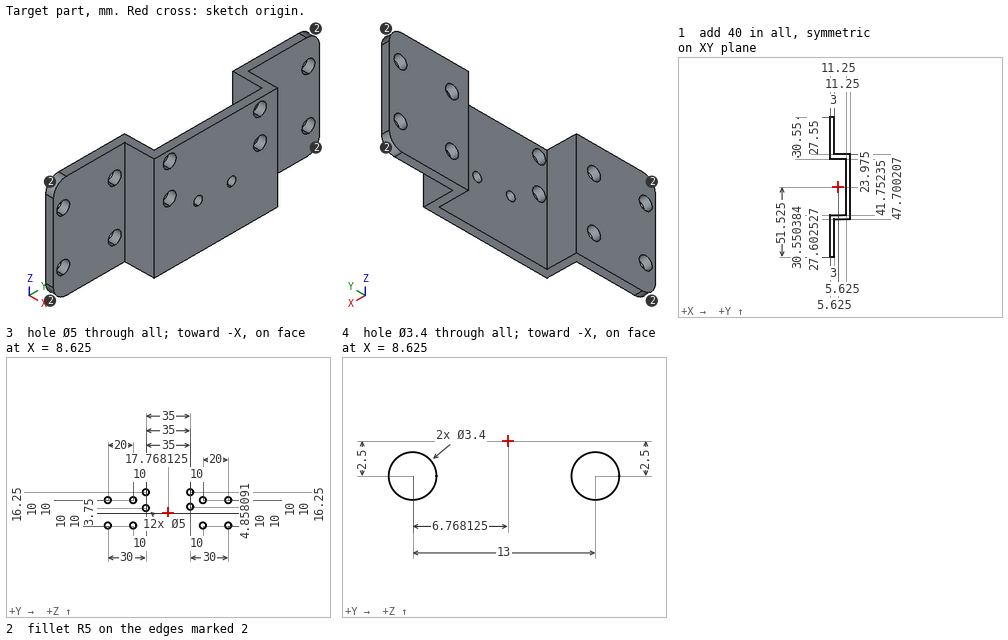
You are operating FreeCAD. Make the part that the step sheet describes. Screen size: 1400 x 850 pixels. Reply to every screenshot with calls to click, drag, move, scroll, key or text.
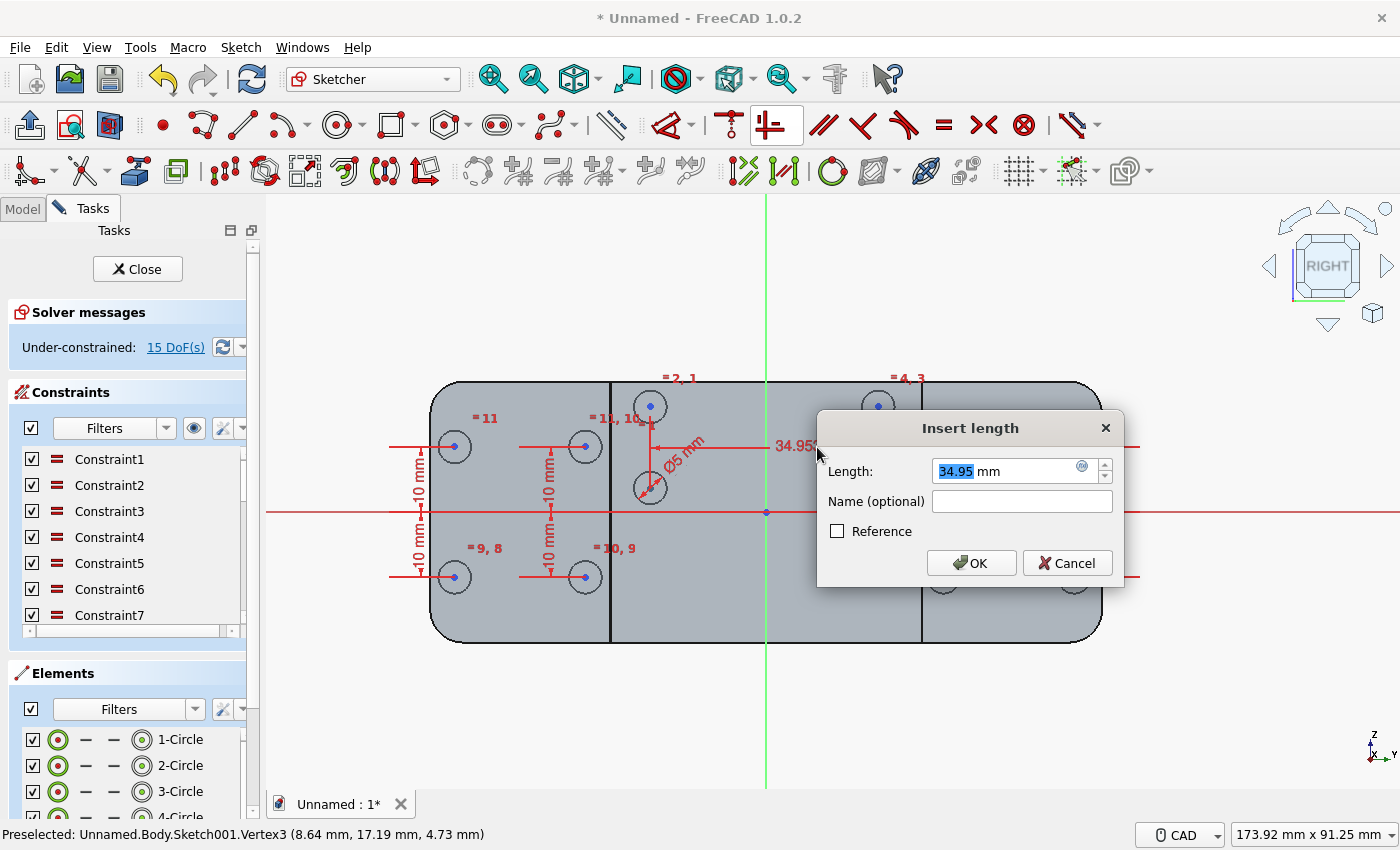
text(35)
key(Return)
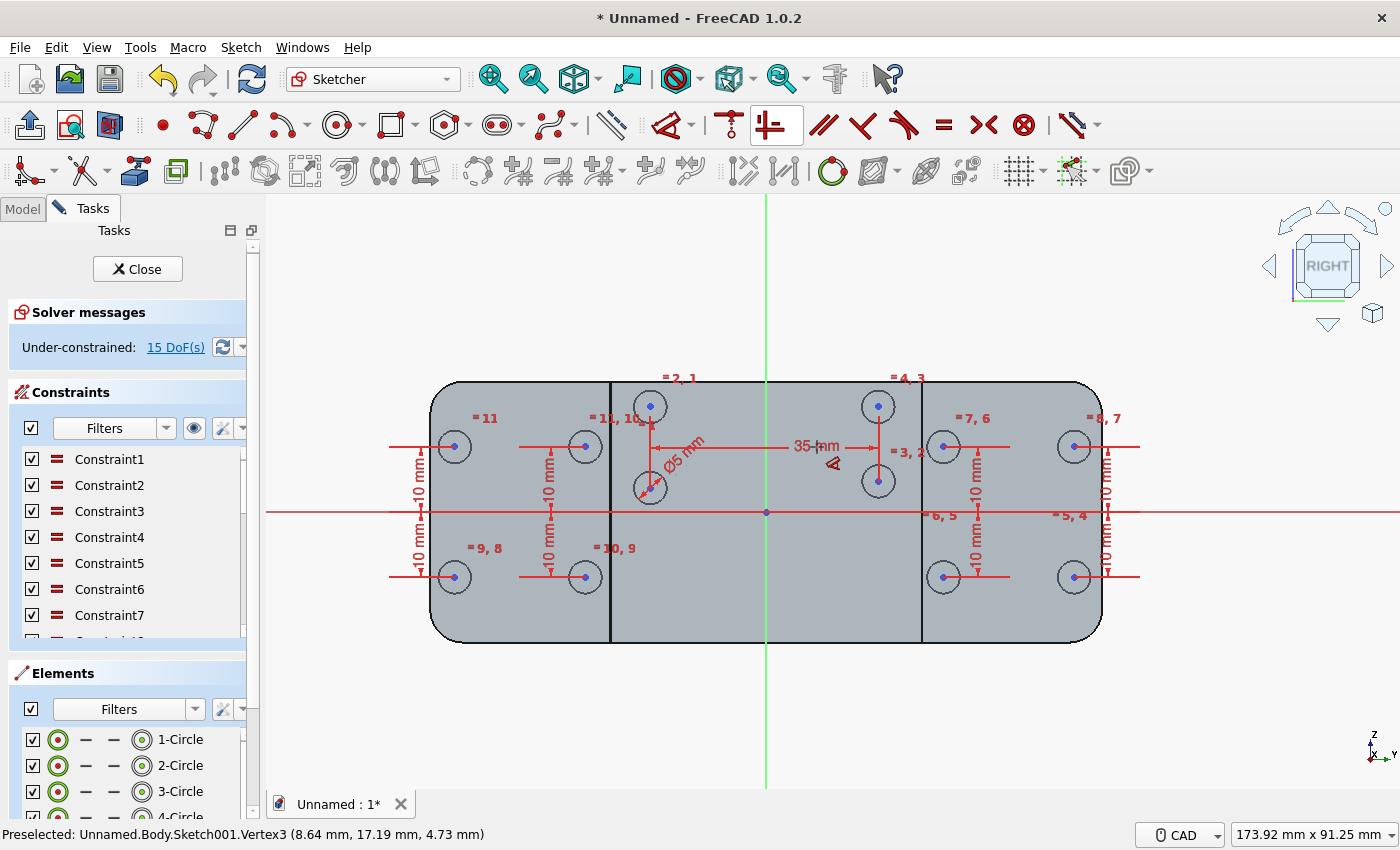
click(650, 407)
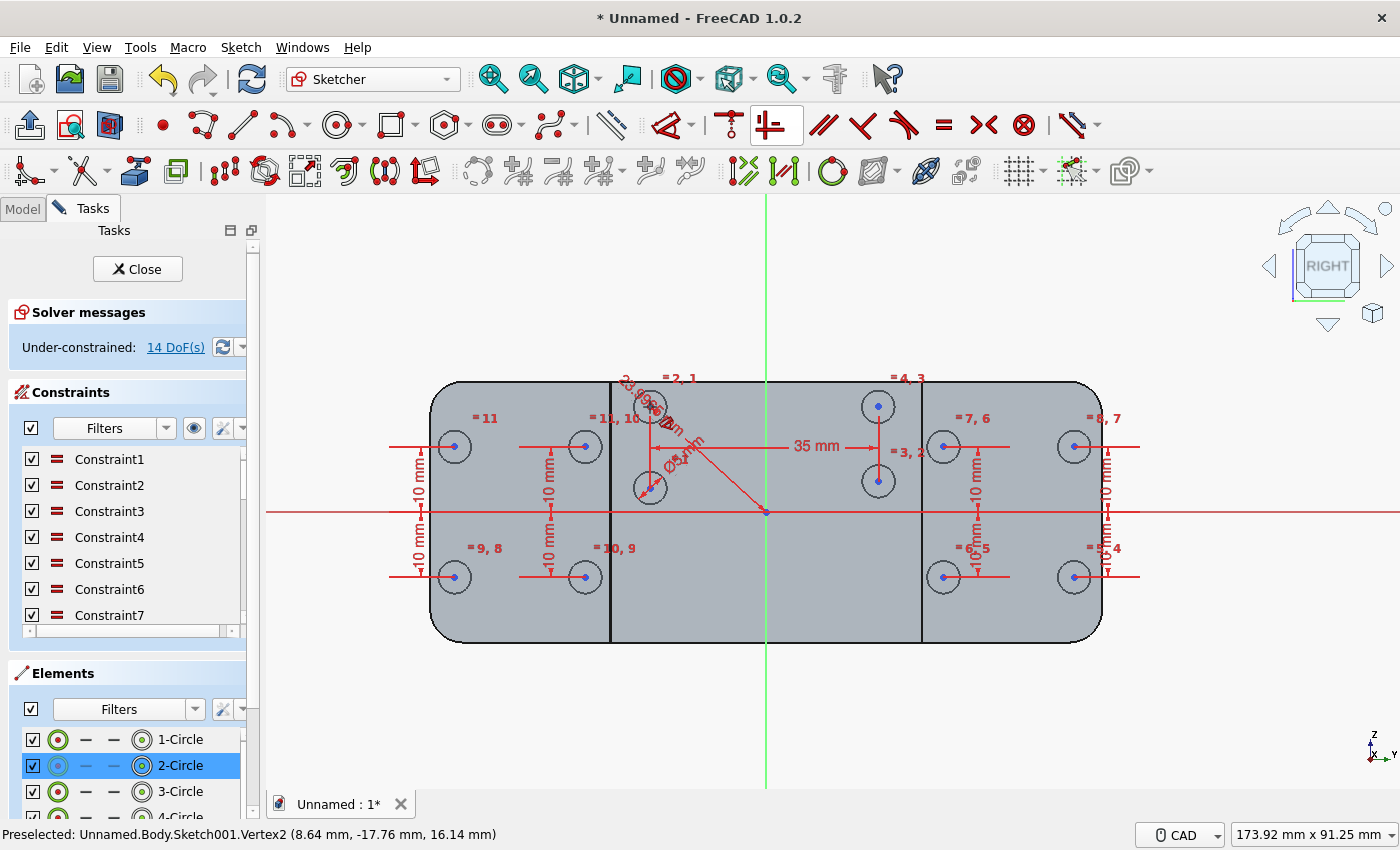
click(879, 481)
click(712, 373)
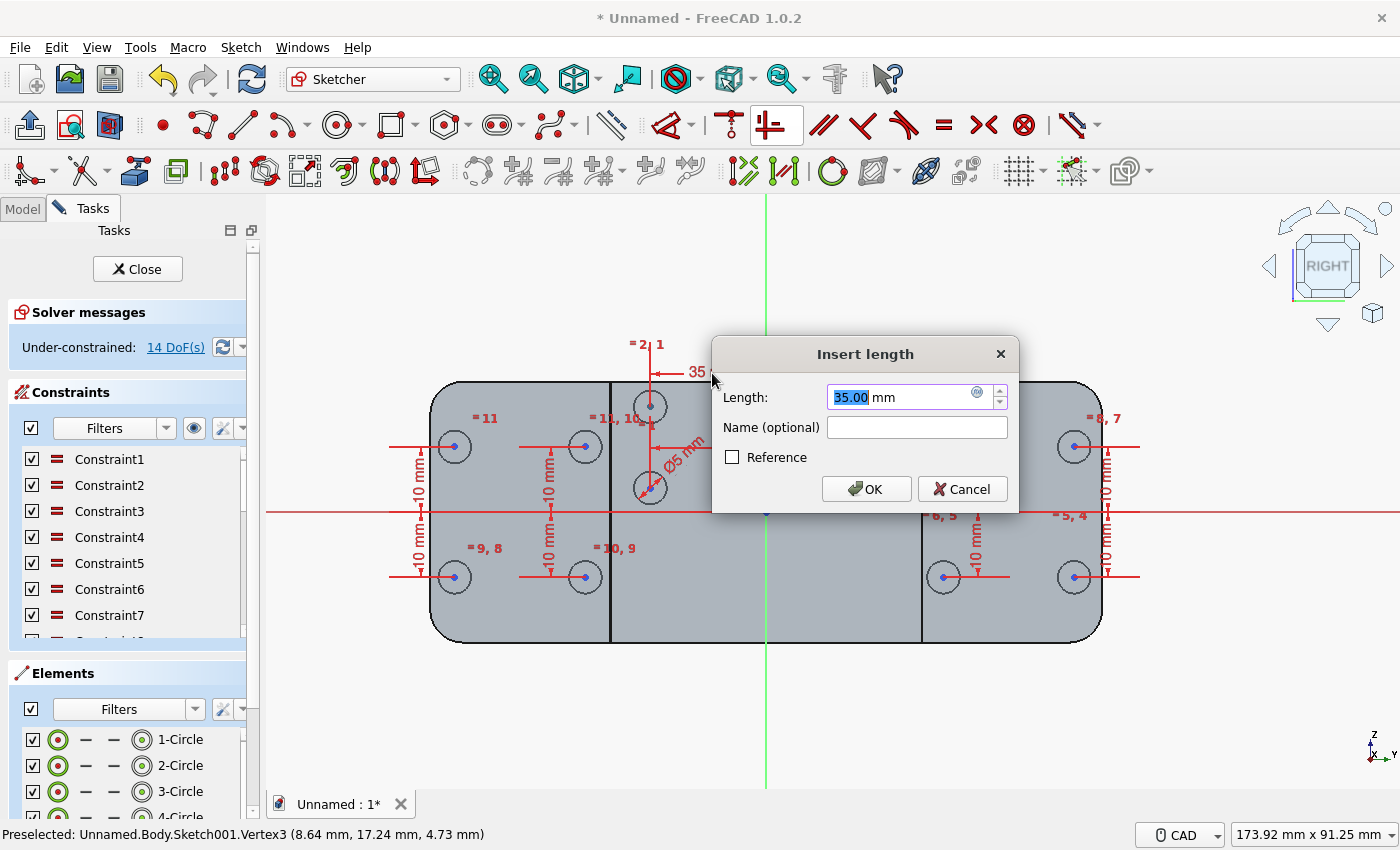
text(35)
key(Return)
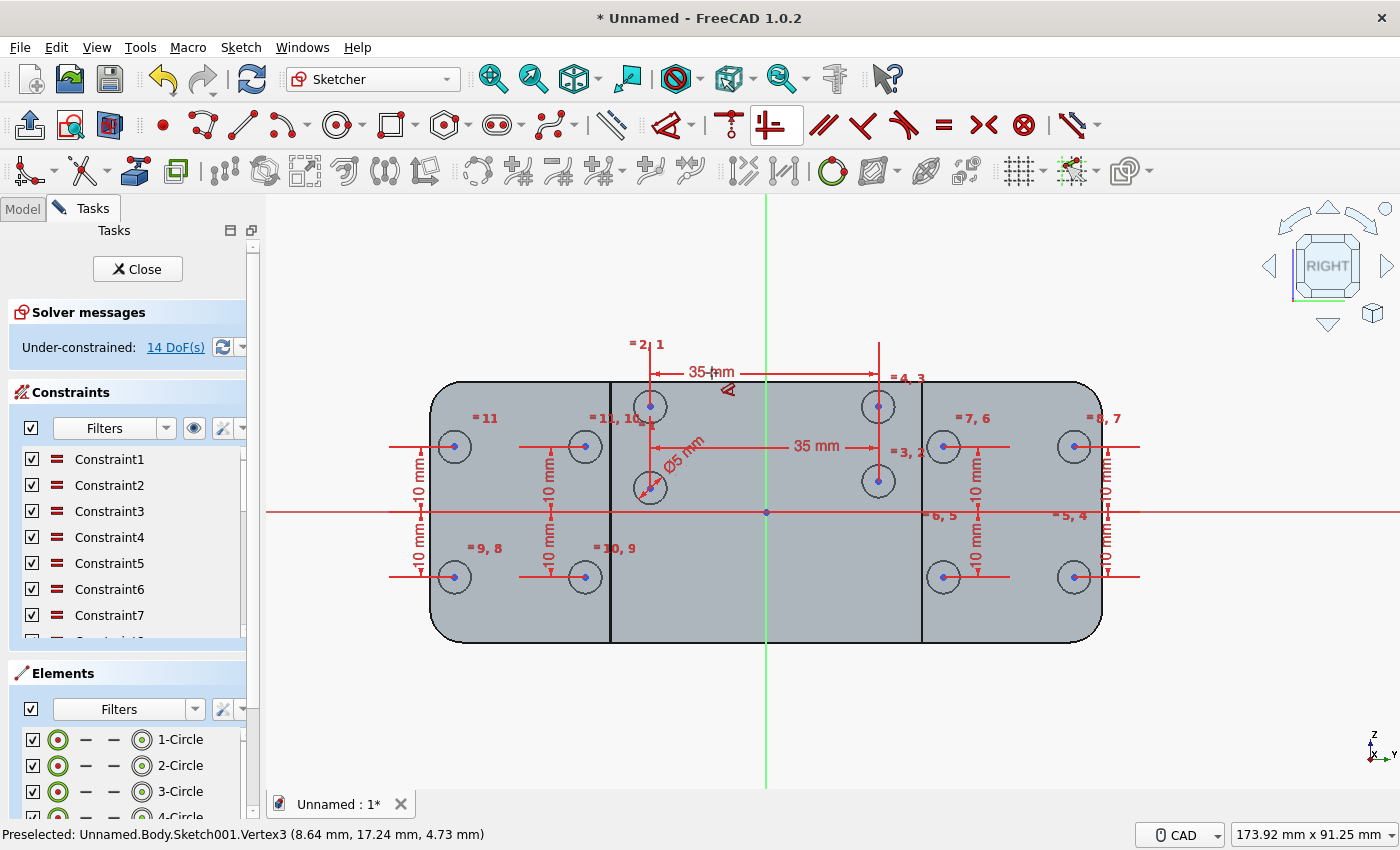
click(650, 407)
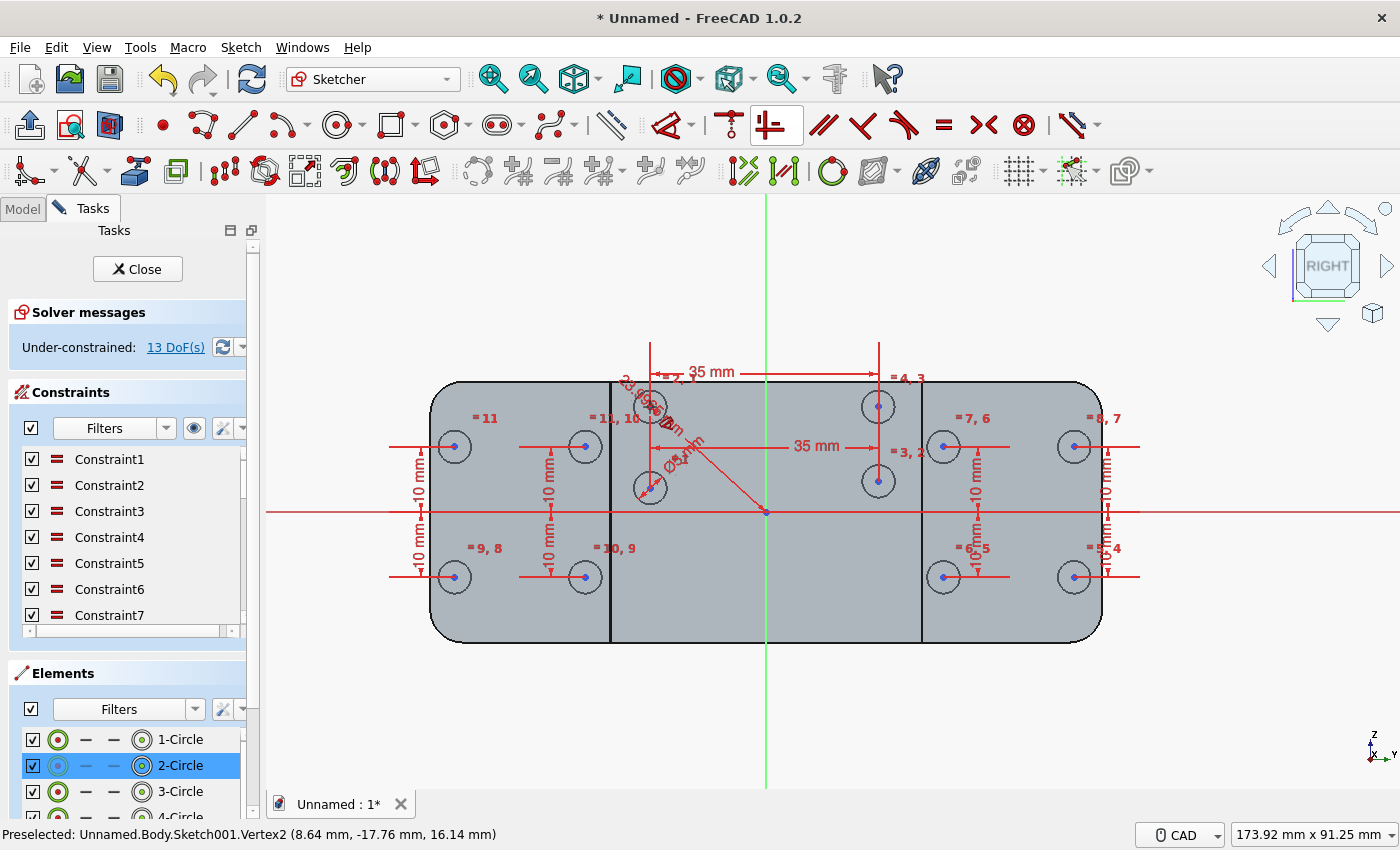
click(878, 407)
click(817, 373)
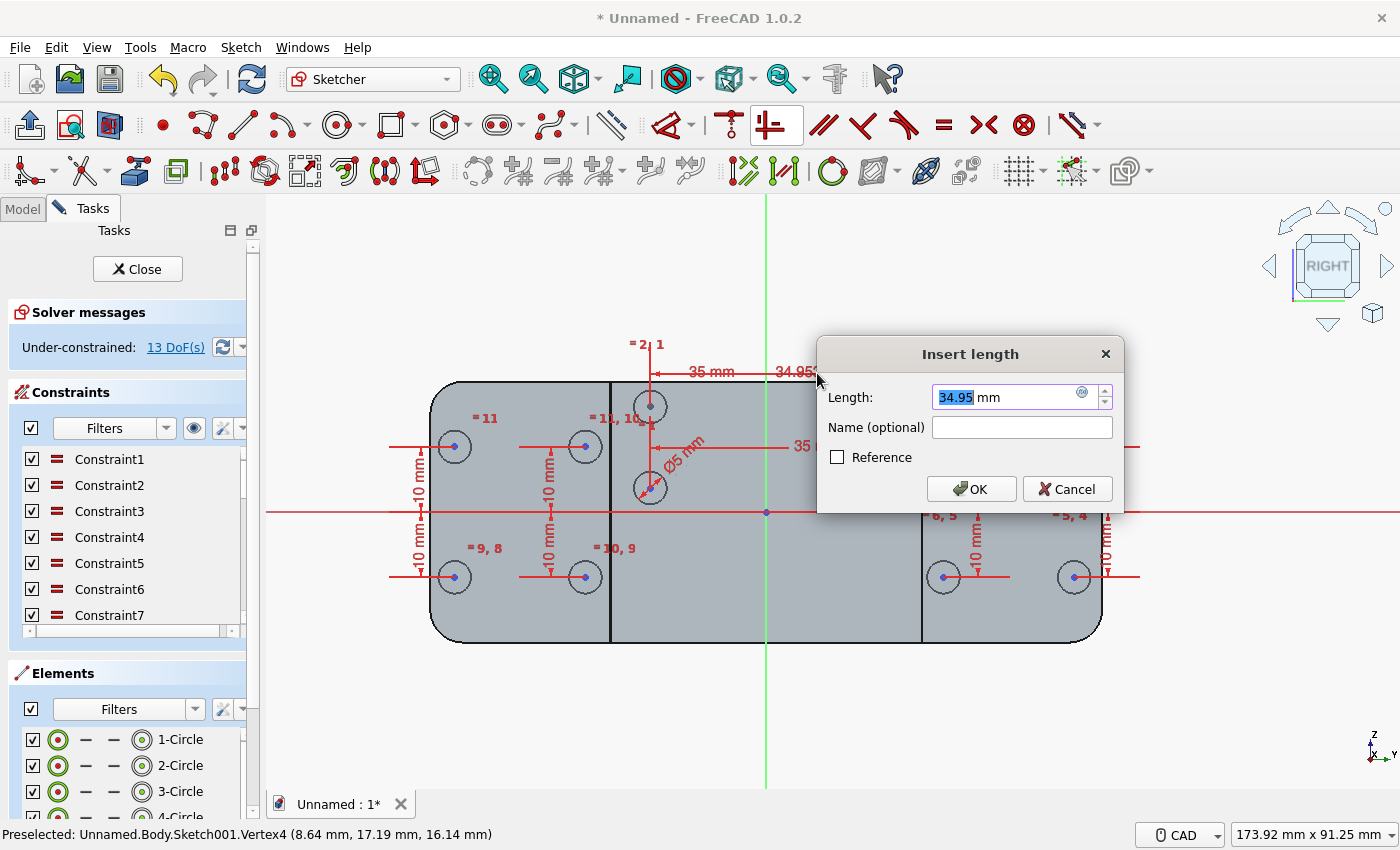
text(35)
key(Return)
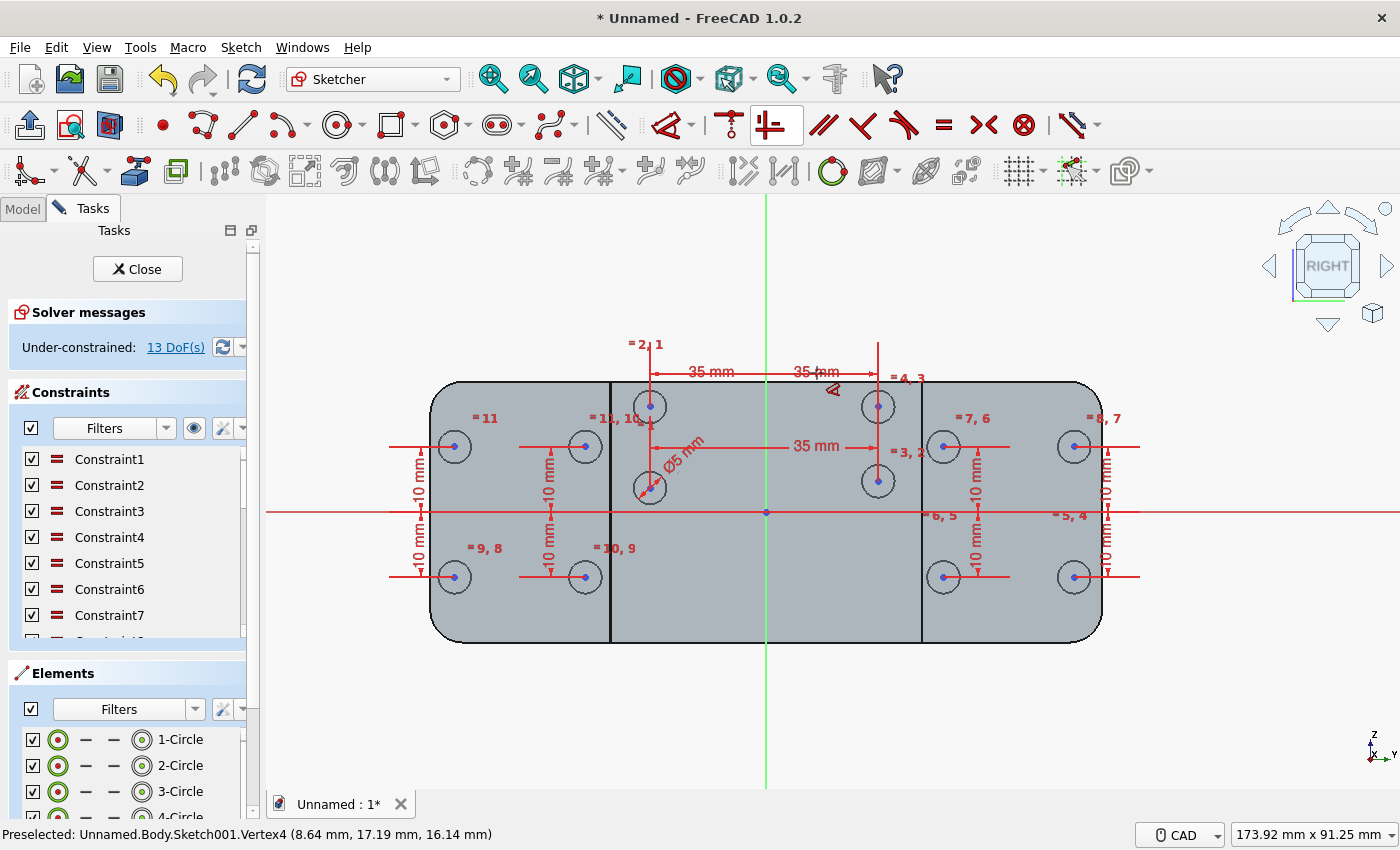
click(878, 481)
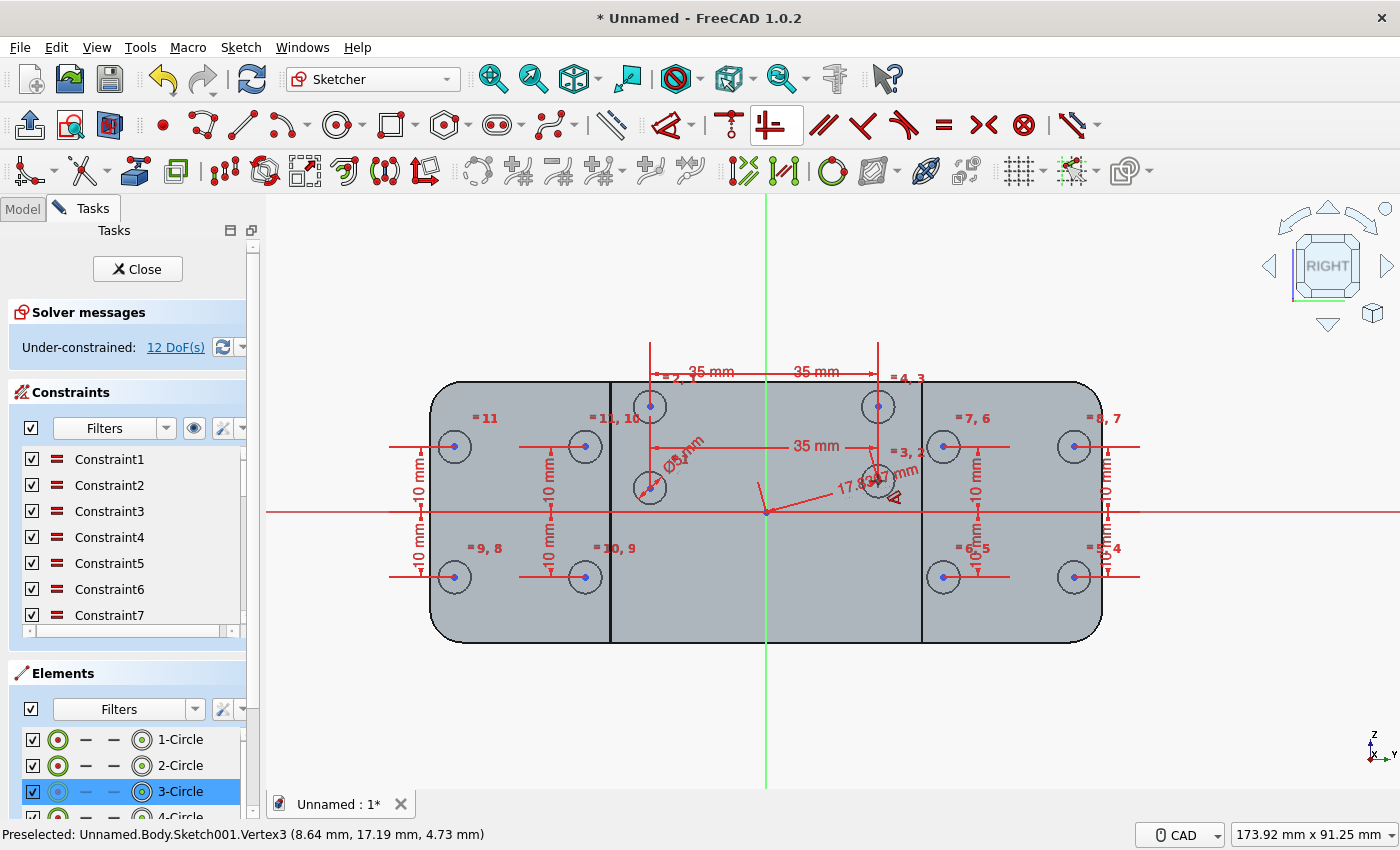
click(1074, 577)
click(976, 611)